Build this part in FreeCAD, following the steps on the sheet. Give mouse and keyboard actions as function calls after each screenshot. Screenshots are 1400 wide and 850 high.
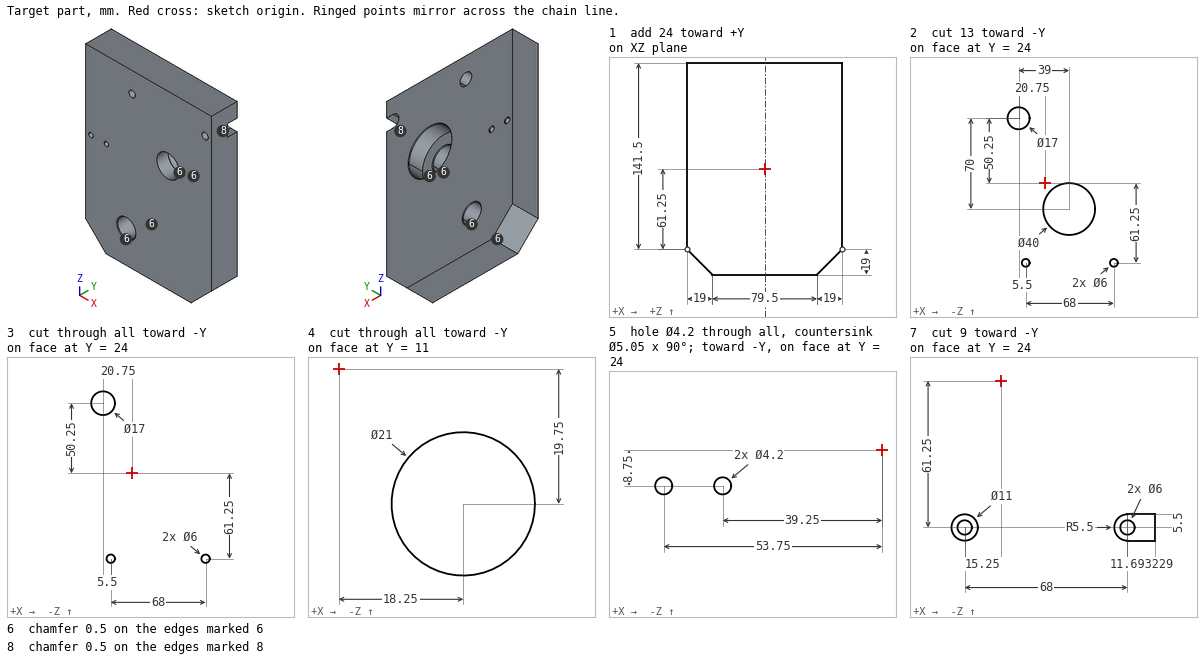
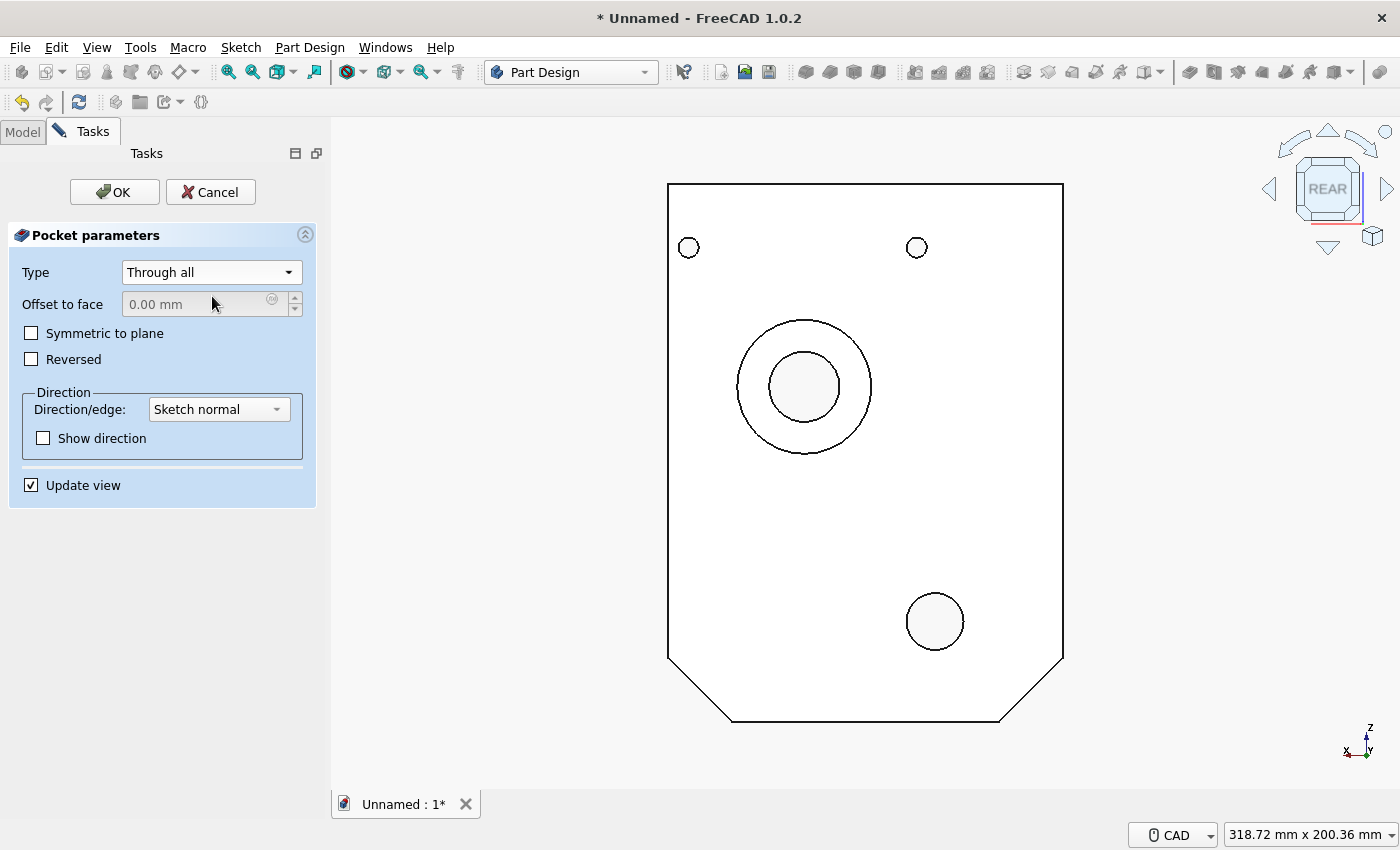
click(115, 192)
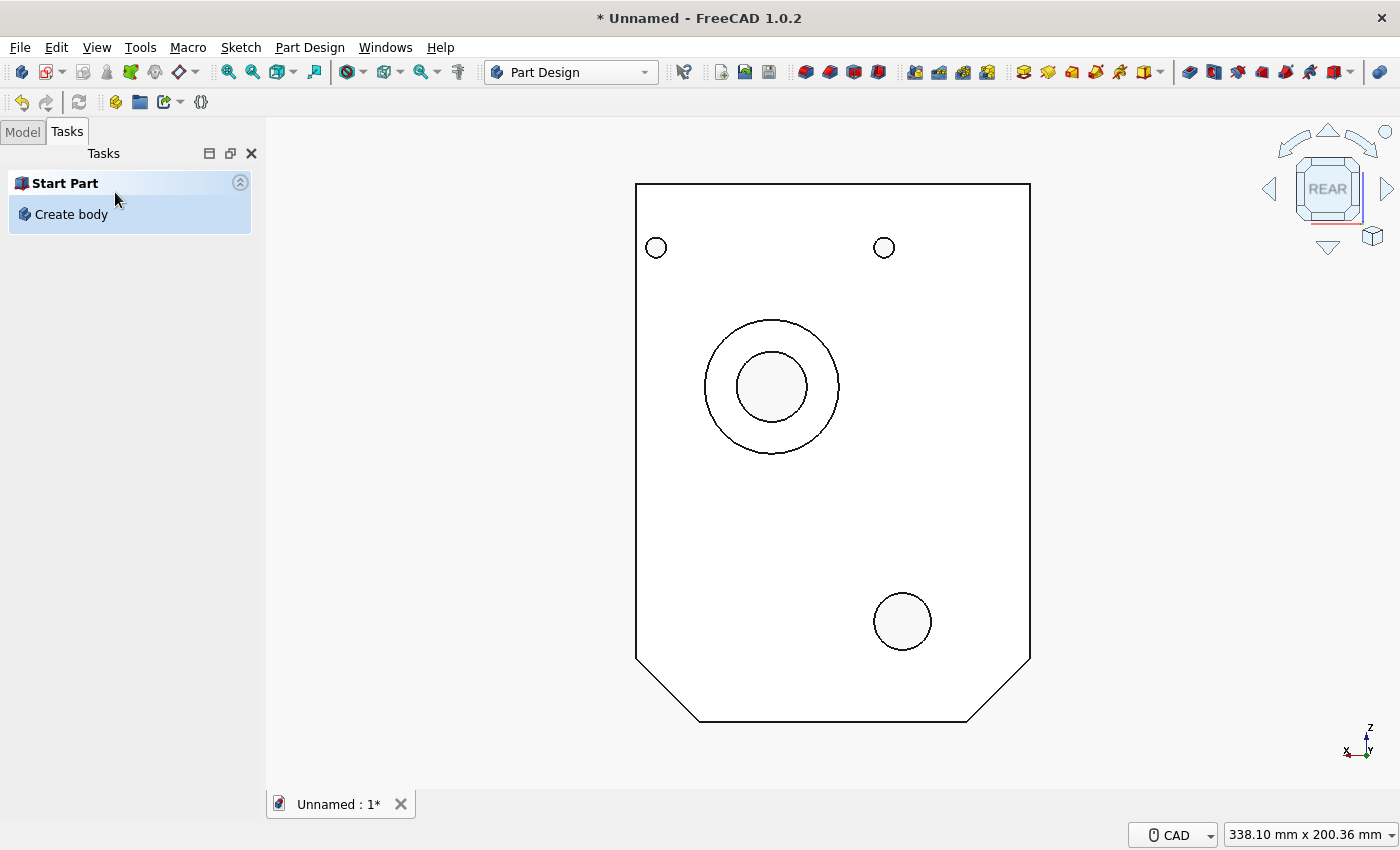
click(777, 606)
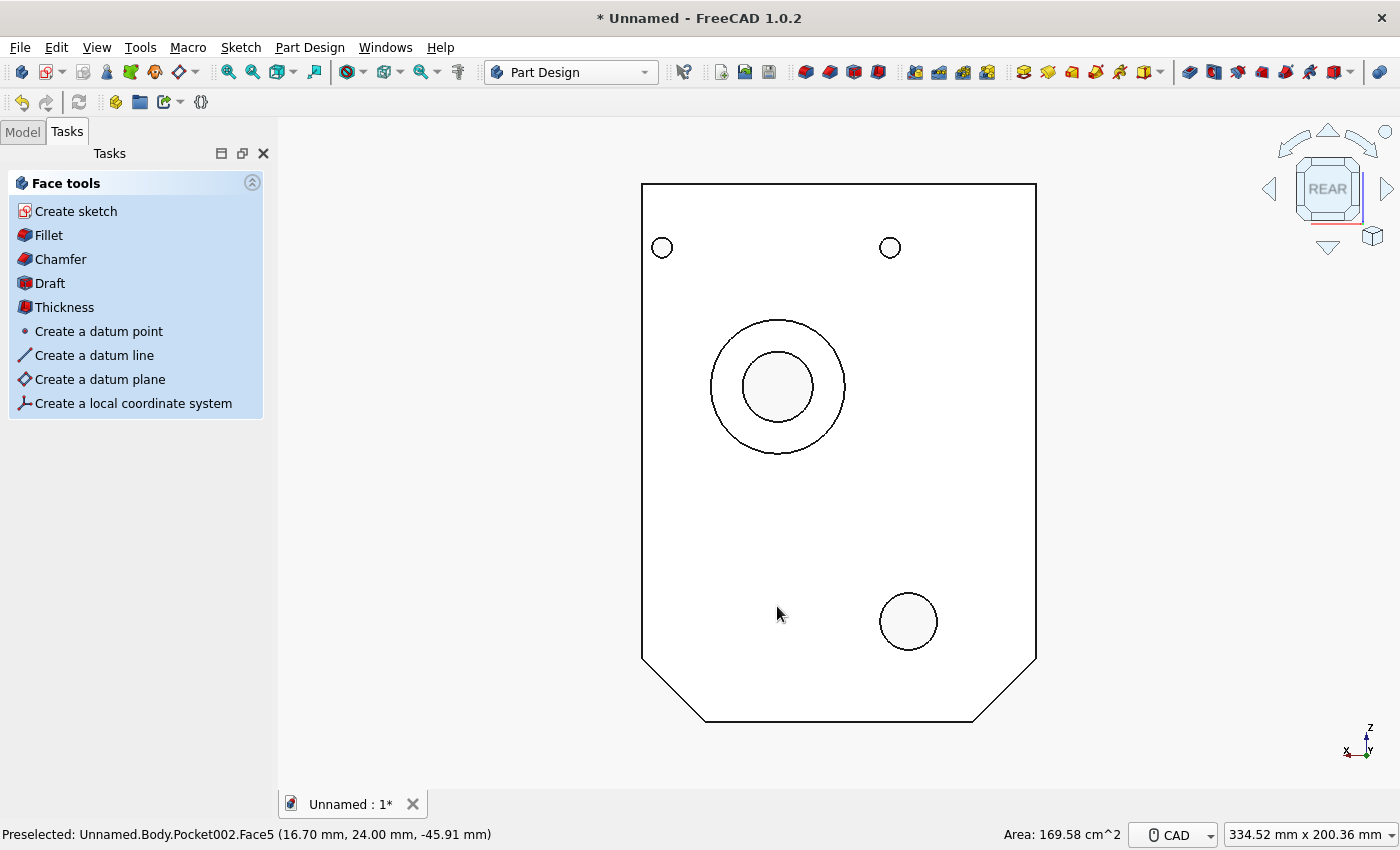
click(46, 72)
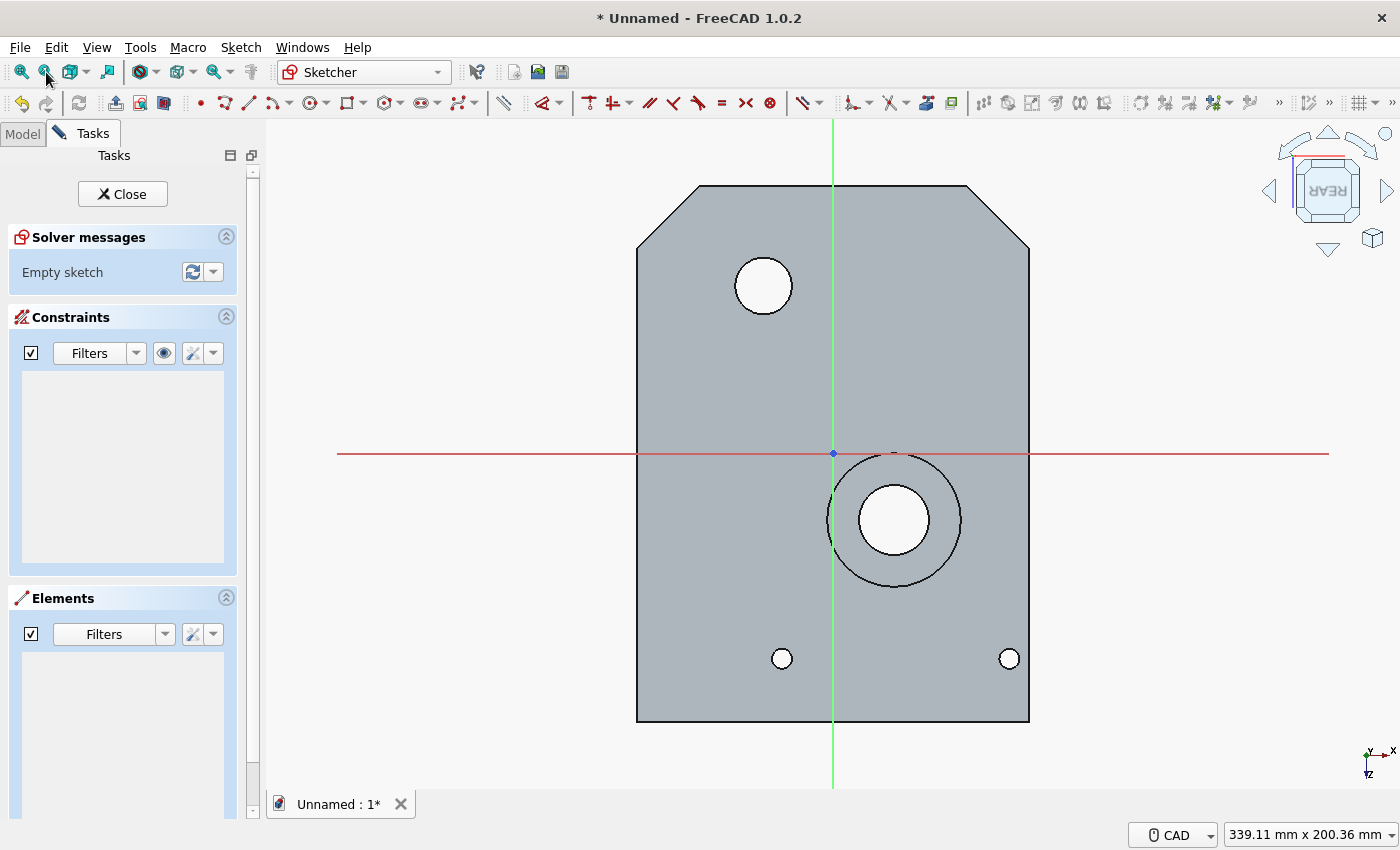
scroll(669, 486, up, 12)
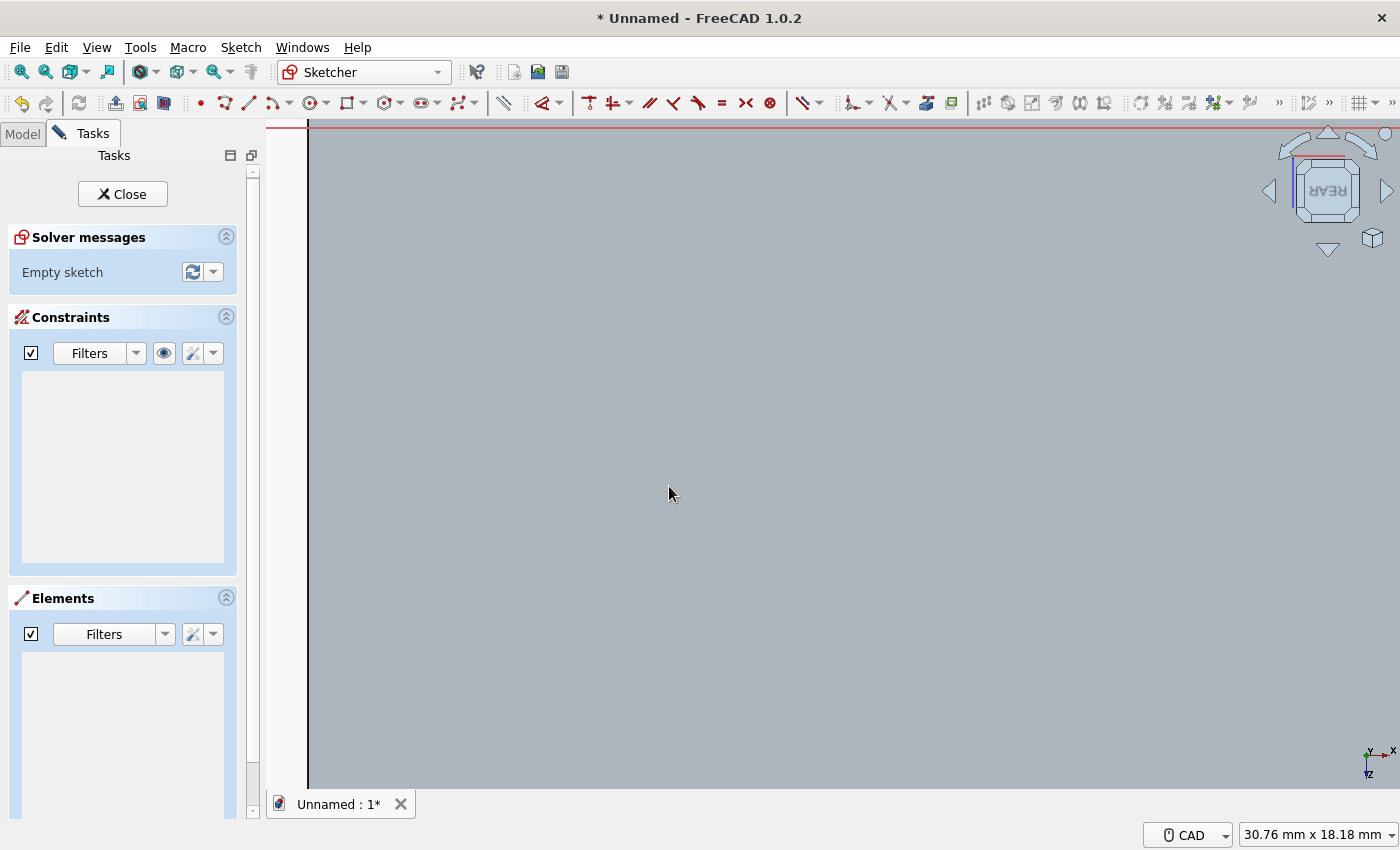
key(g)
key(c)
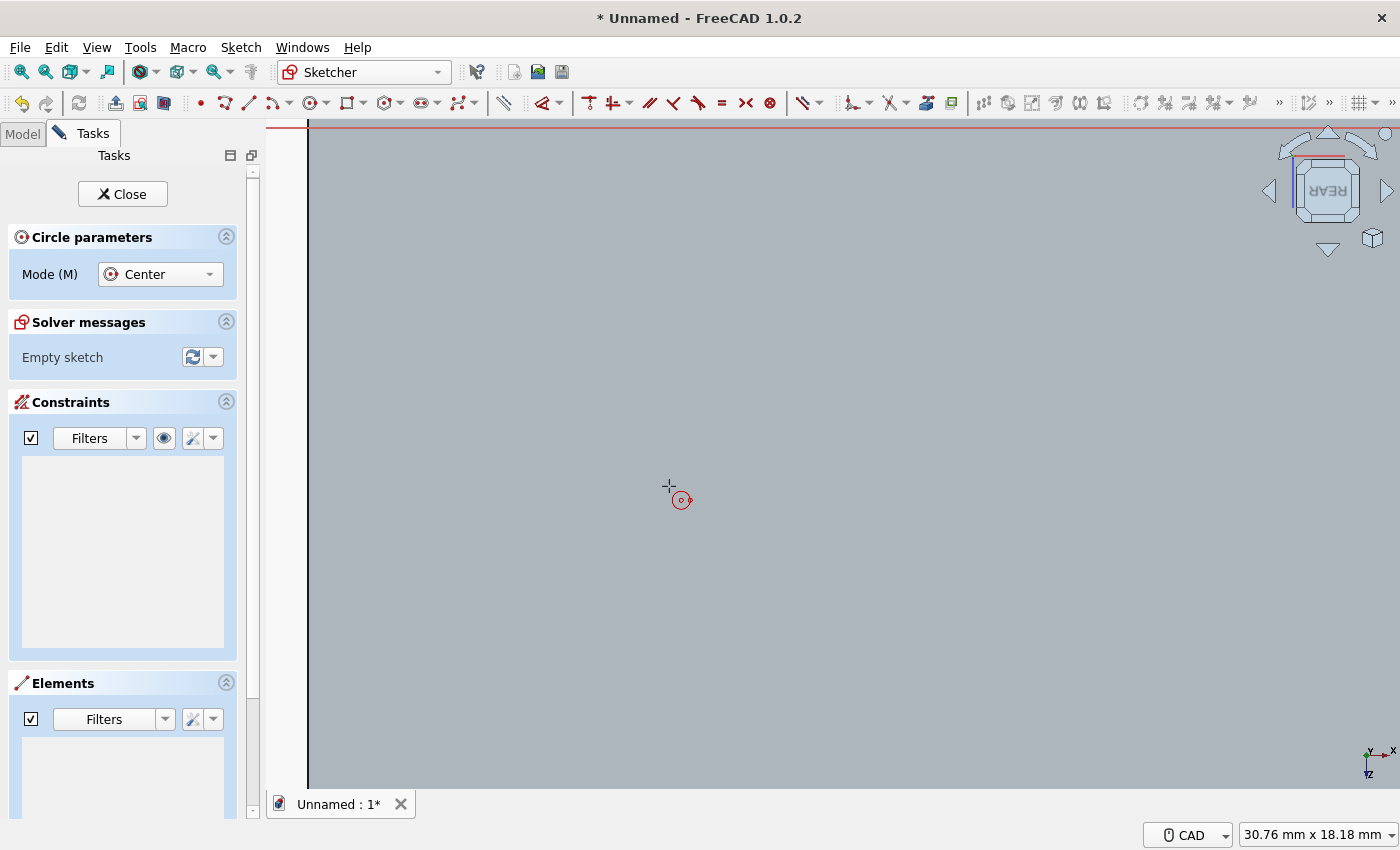
click(1026, 450)
move(1081, 396)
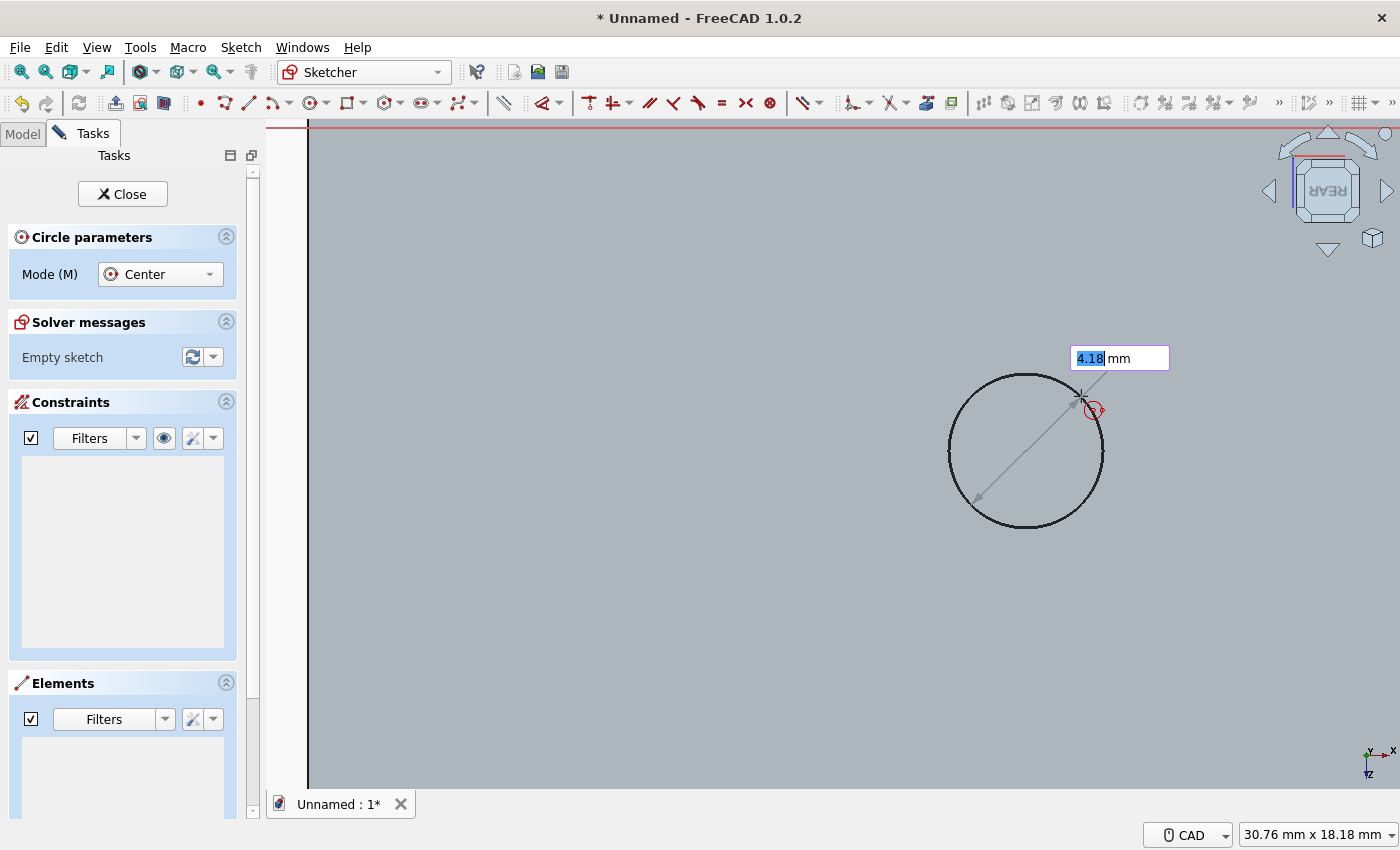
text(4.2)
key(Return)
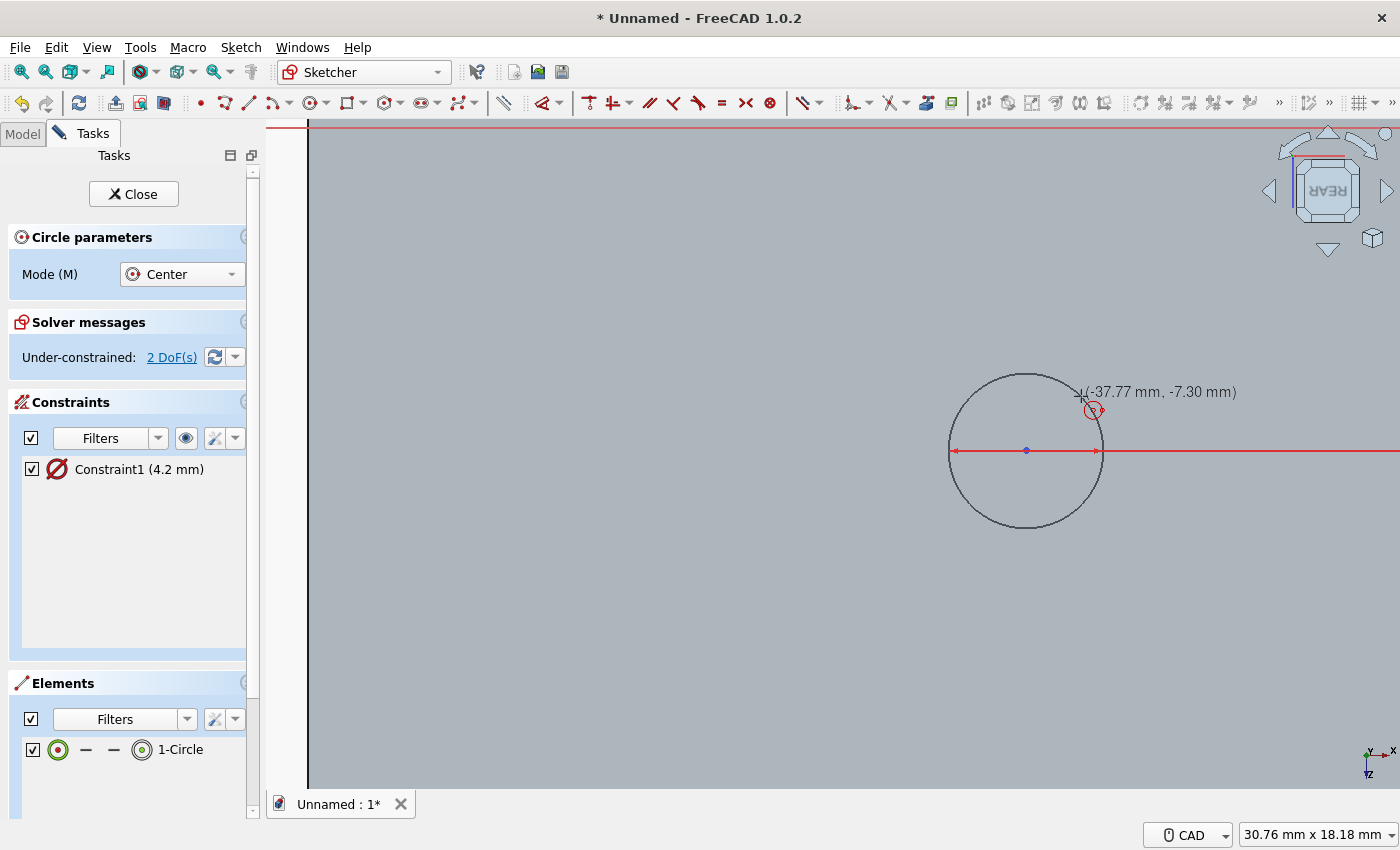
click(492, 450)
move(547, 396)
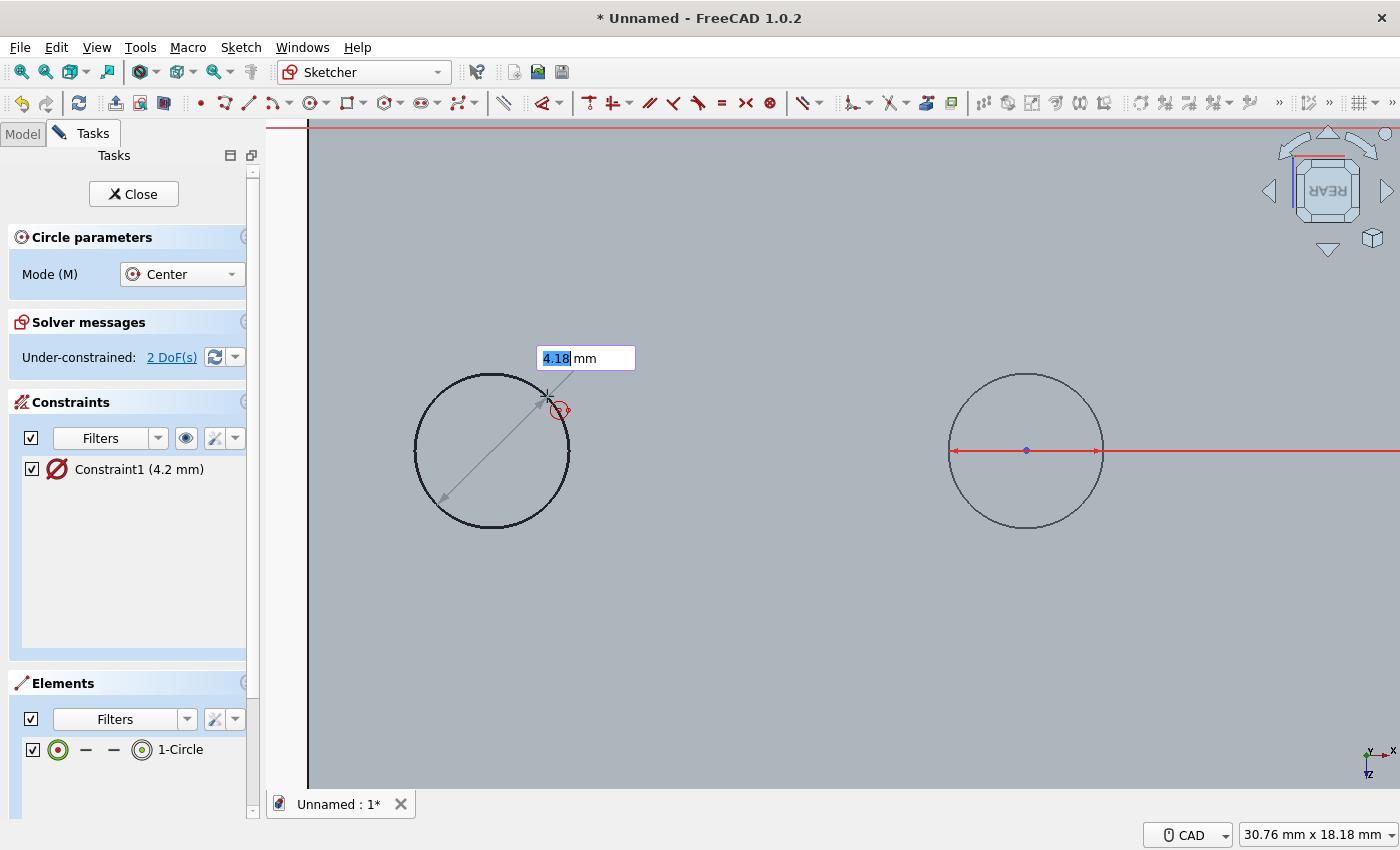
text(4.2)
key(Return)
key(Escape)